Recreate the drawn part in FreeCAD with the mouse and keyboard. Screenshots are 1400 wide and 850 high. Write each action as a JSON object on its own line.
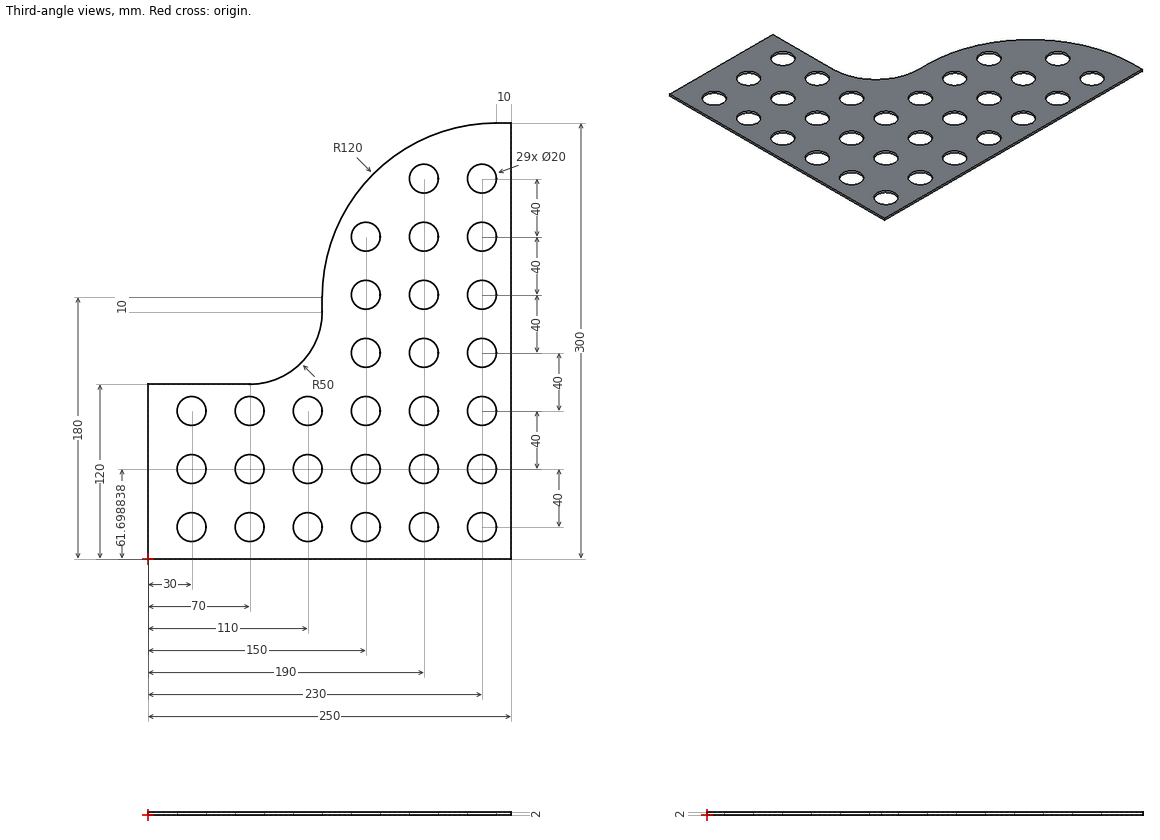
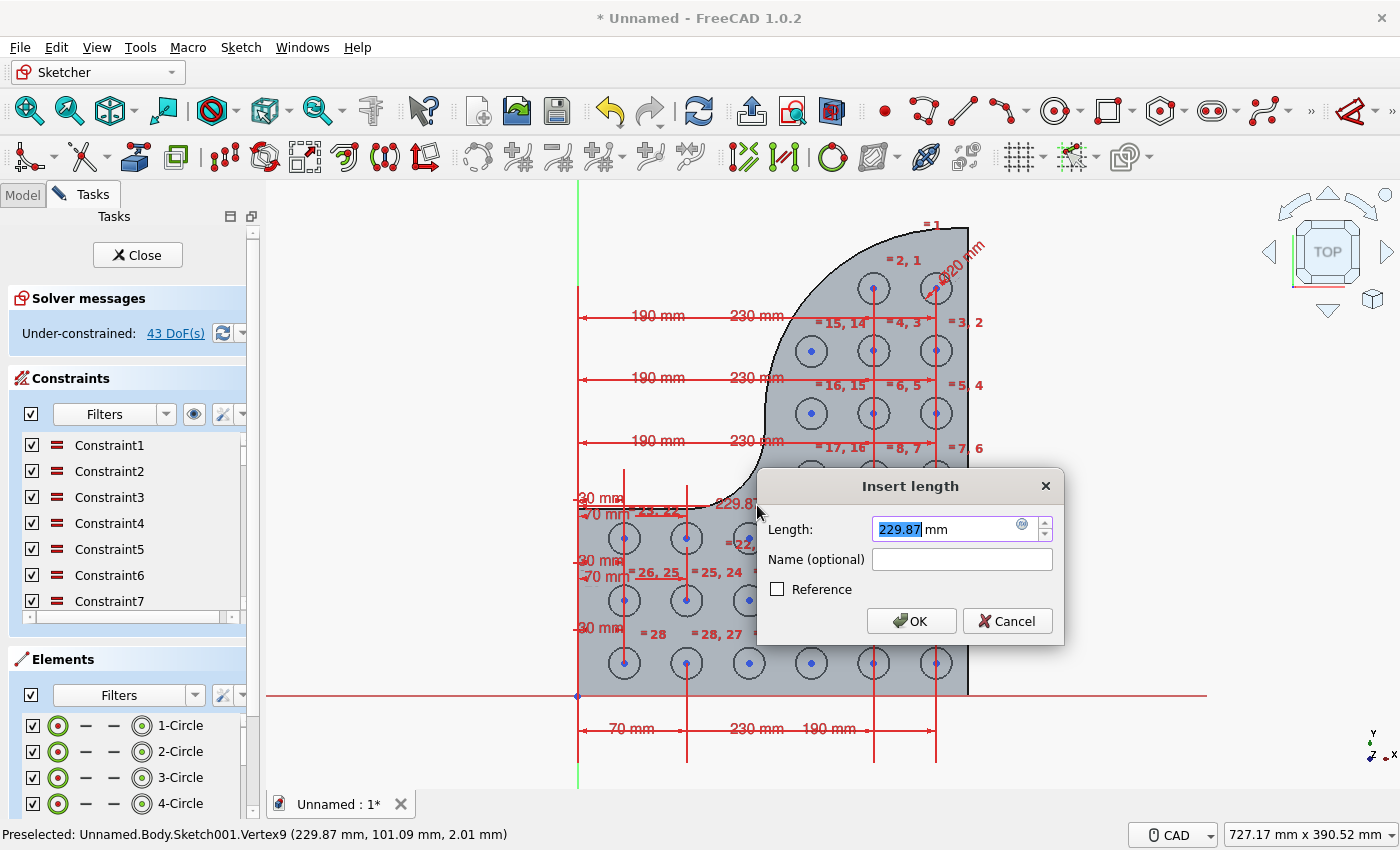
{"action": "type", "text": "230"}
{"action": "key", "text": "Return"}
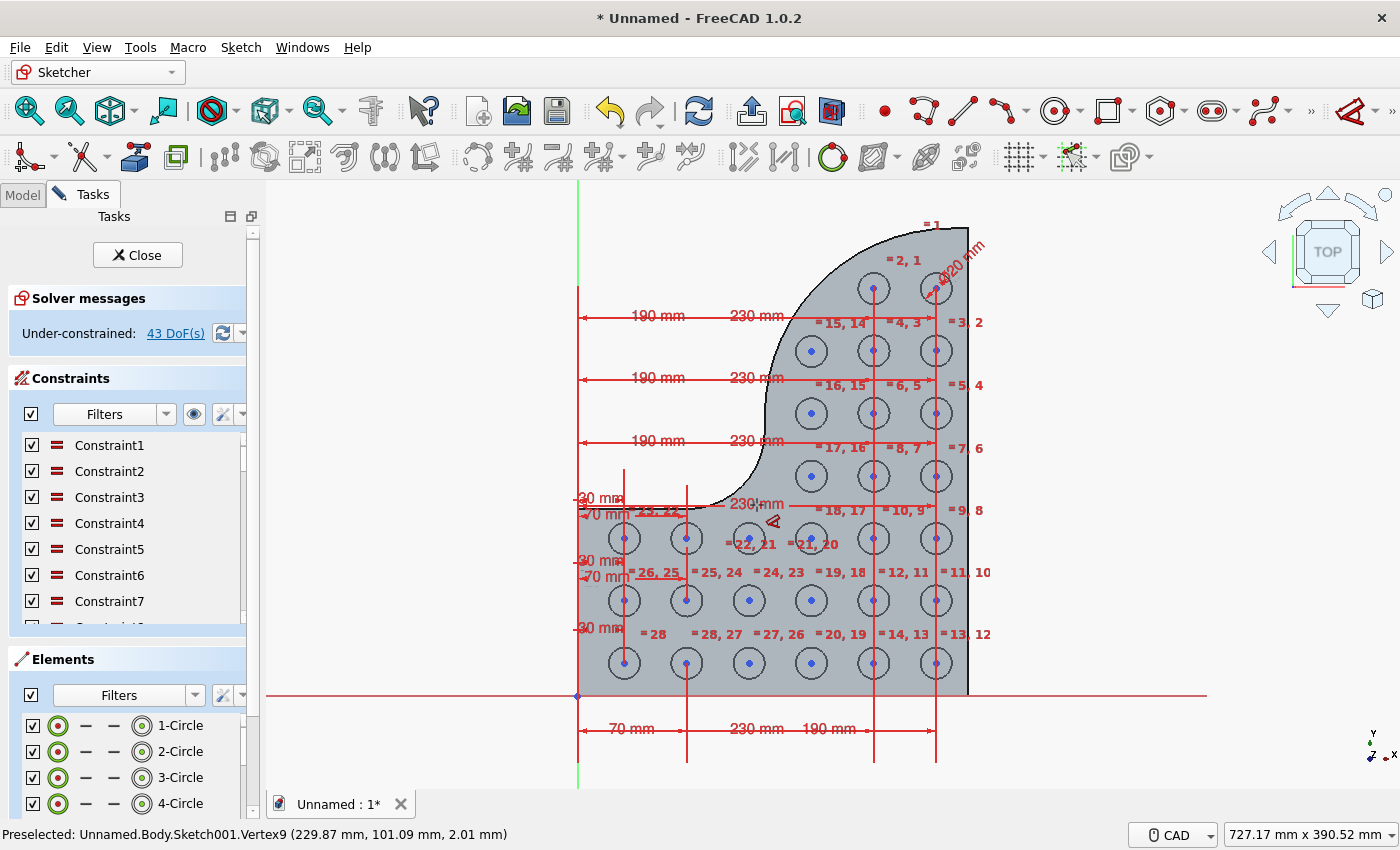
{"action": "left_click", "coordinate": [874, 539]}
{"action": "left_click", "coordinate": [829, 505]}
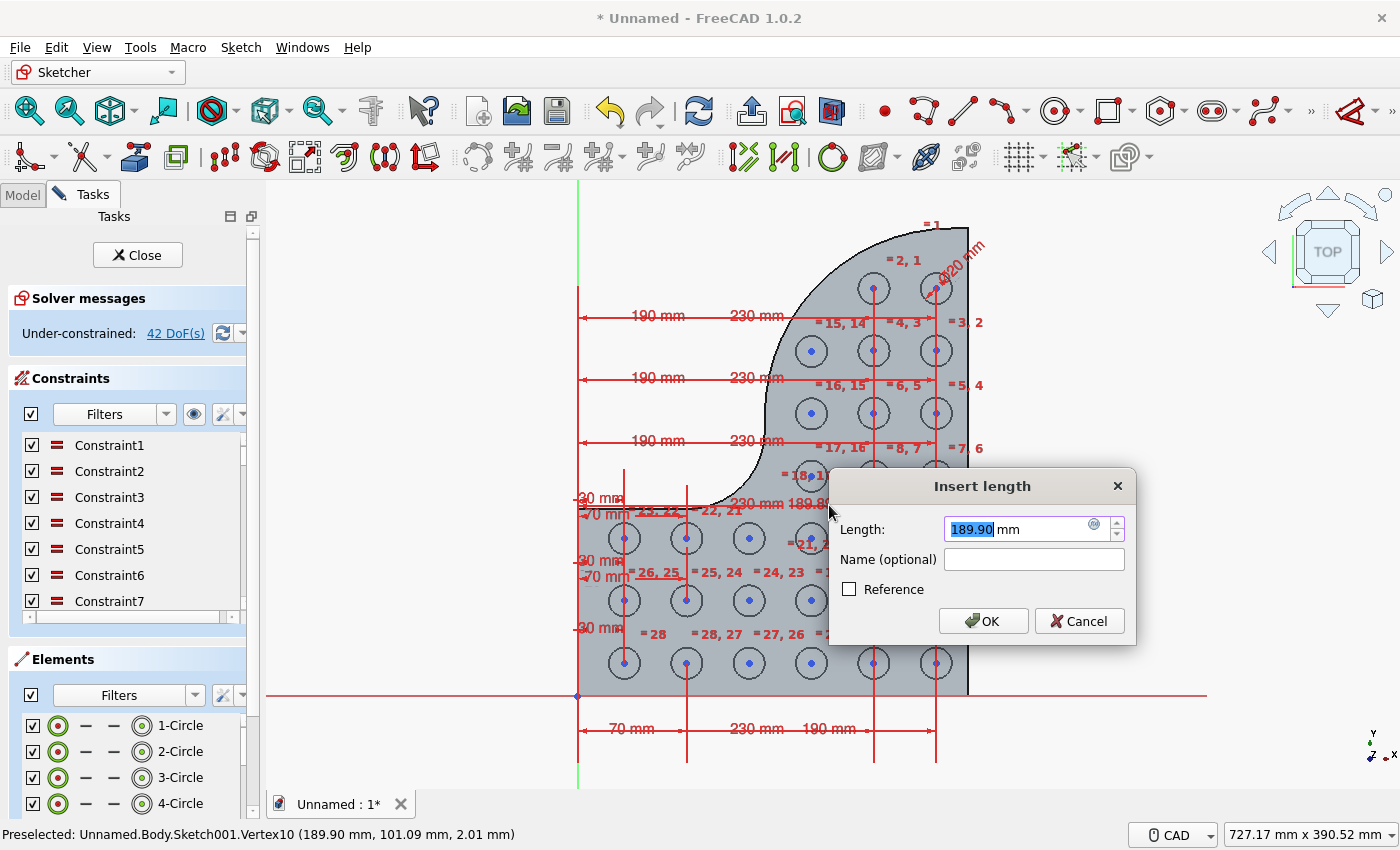
{"action": "type", "text": "190"}
{"action": "key", "text": "Return"}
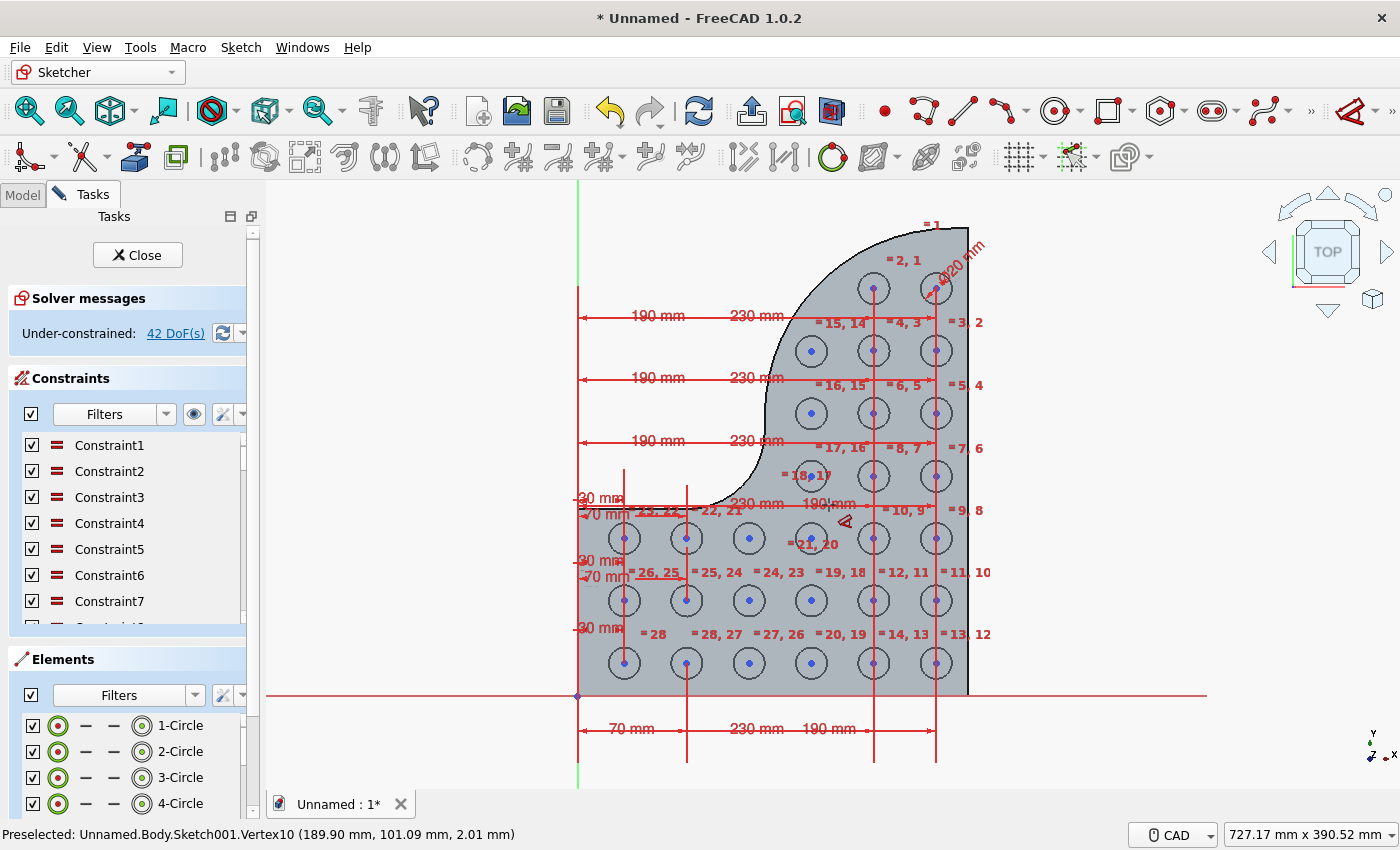
{"action": "left_click", "coordinate": [936, 601]}
{"action": "left_click", "coordinate": [757, 567]}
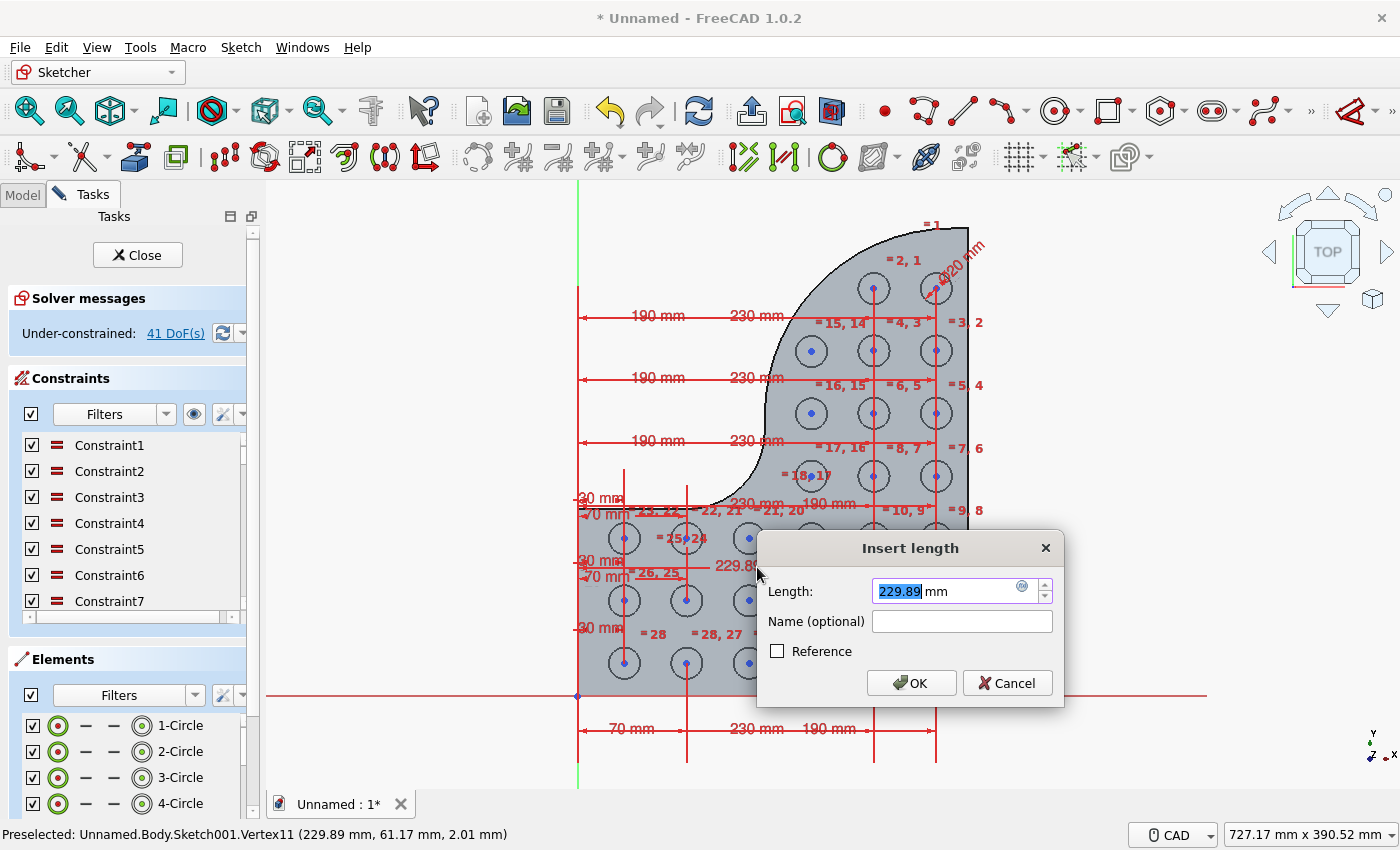
{"action": "type", "text": "230"}
{"action": "key", "text": "Return"}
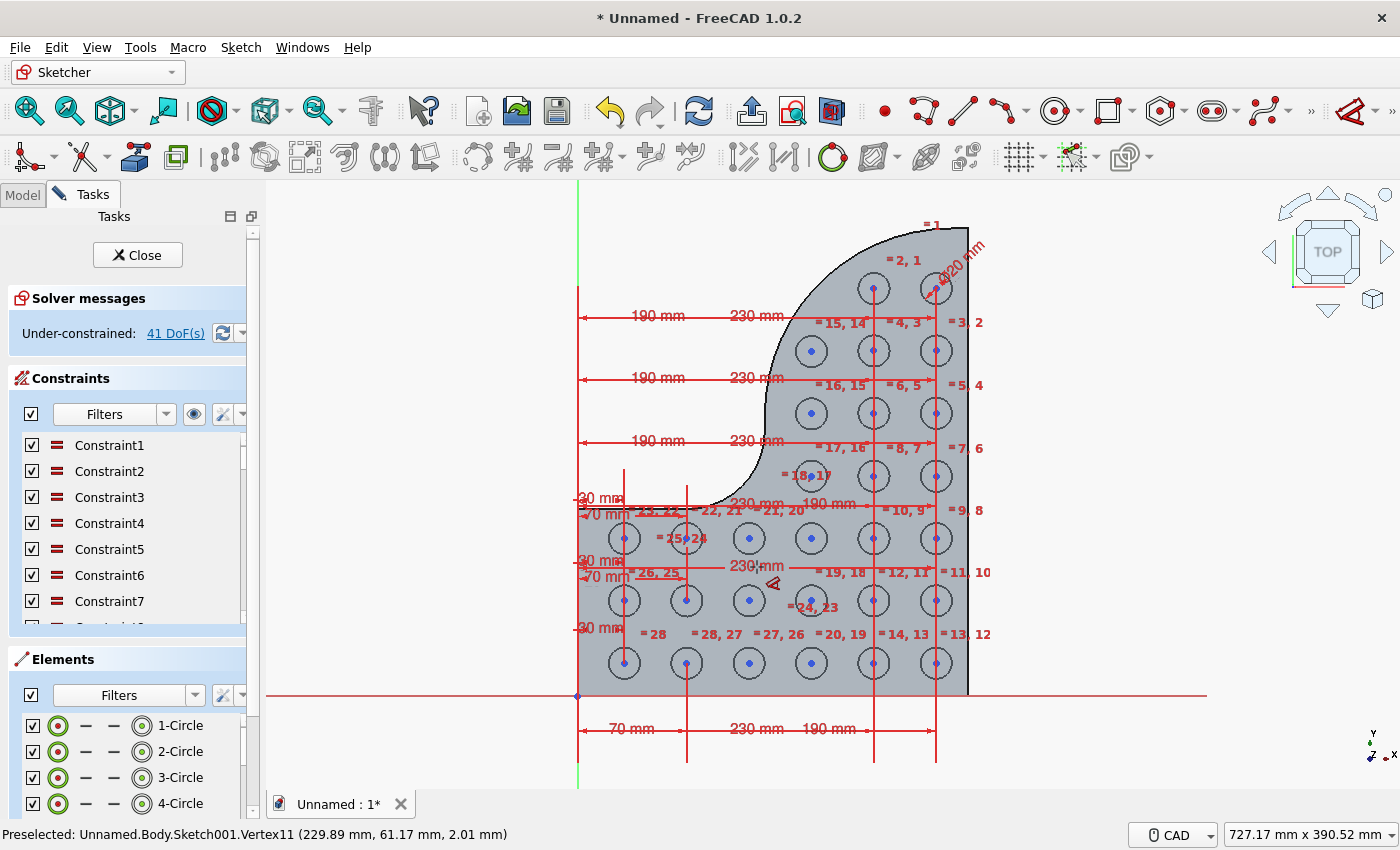
{"action": "left_click", "coordinate": [874, 601]}
{"action": "left_click", "coordinate": [829, 567]}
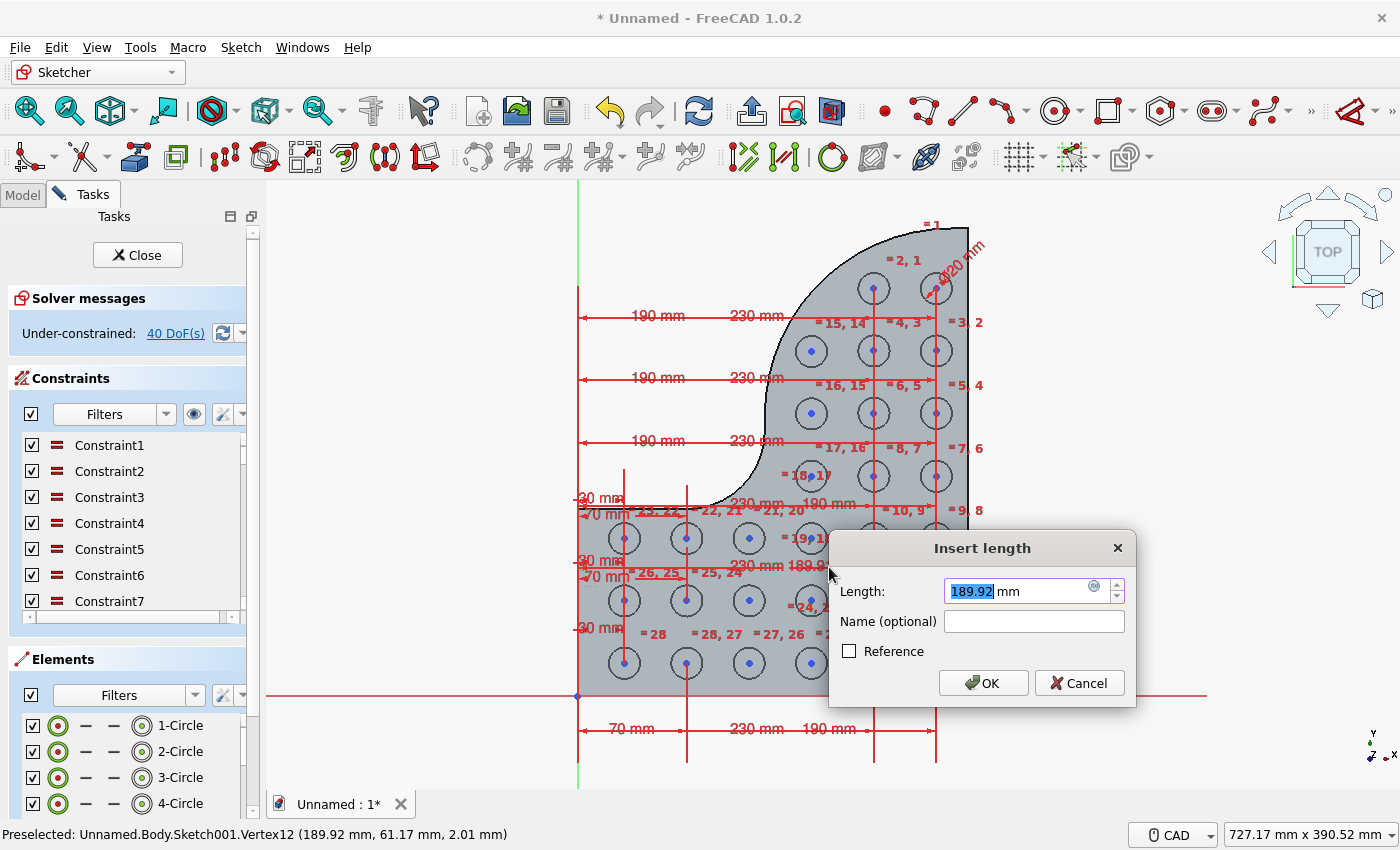
{"action": "type", "text": "190"}
{"action": "key", "text": "Return"}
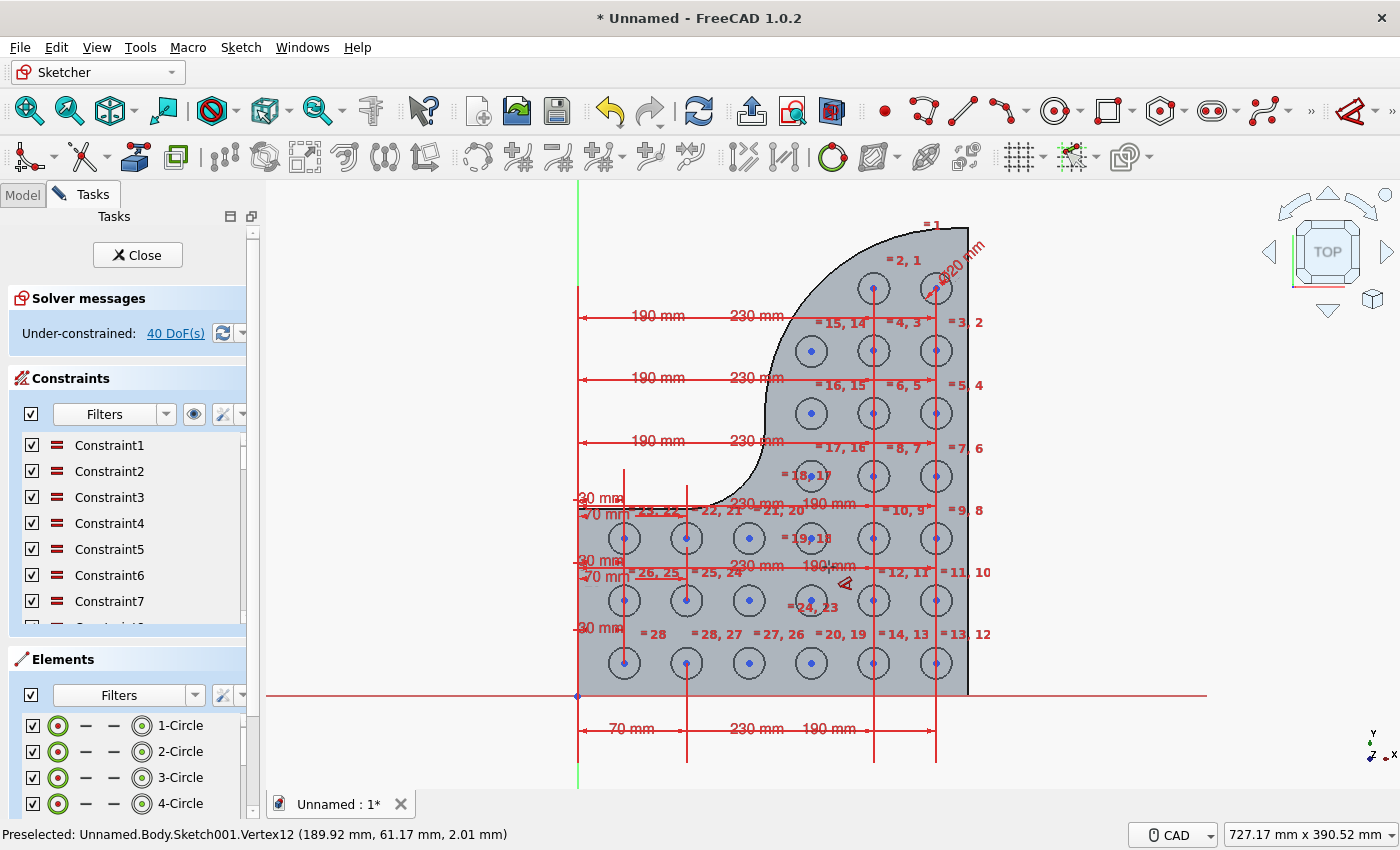
{"action": "left_click", "coordinate": [936, 663]}
{"action": "left_click", "coordinate": [757, 629]}